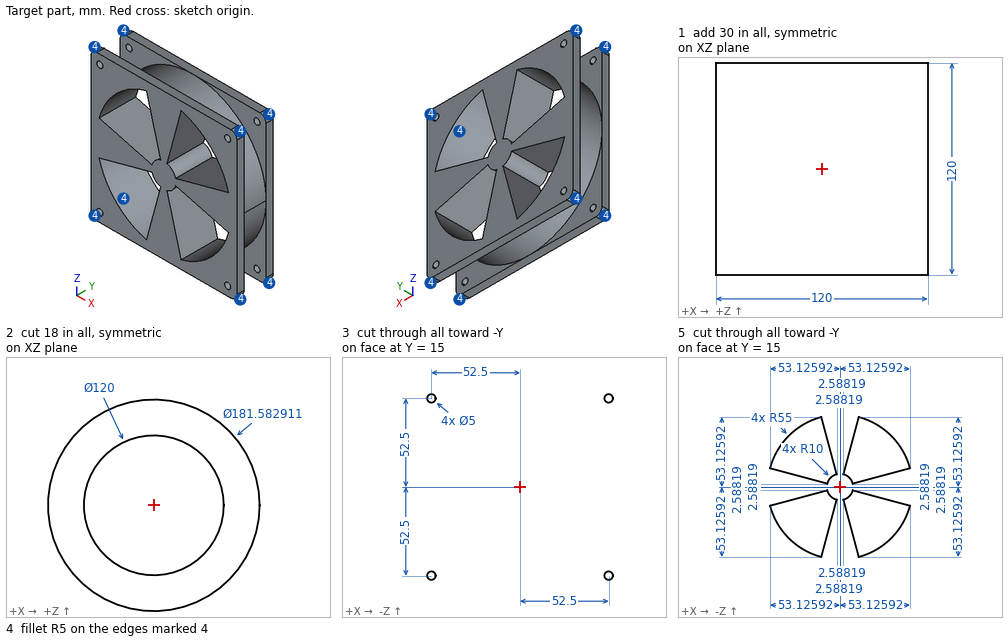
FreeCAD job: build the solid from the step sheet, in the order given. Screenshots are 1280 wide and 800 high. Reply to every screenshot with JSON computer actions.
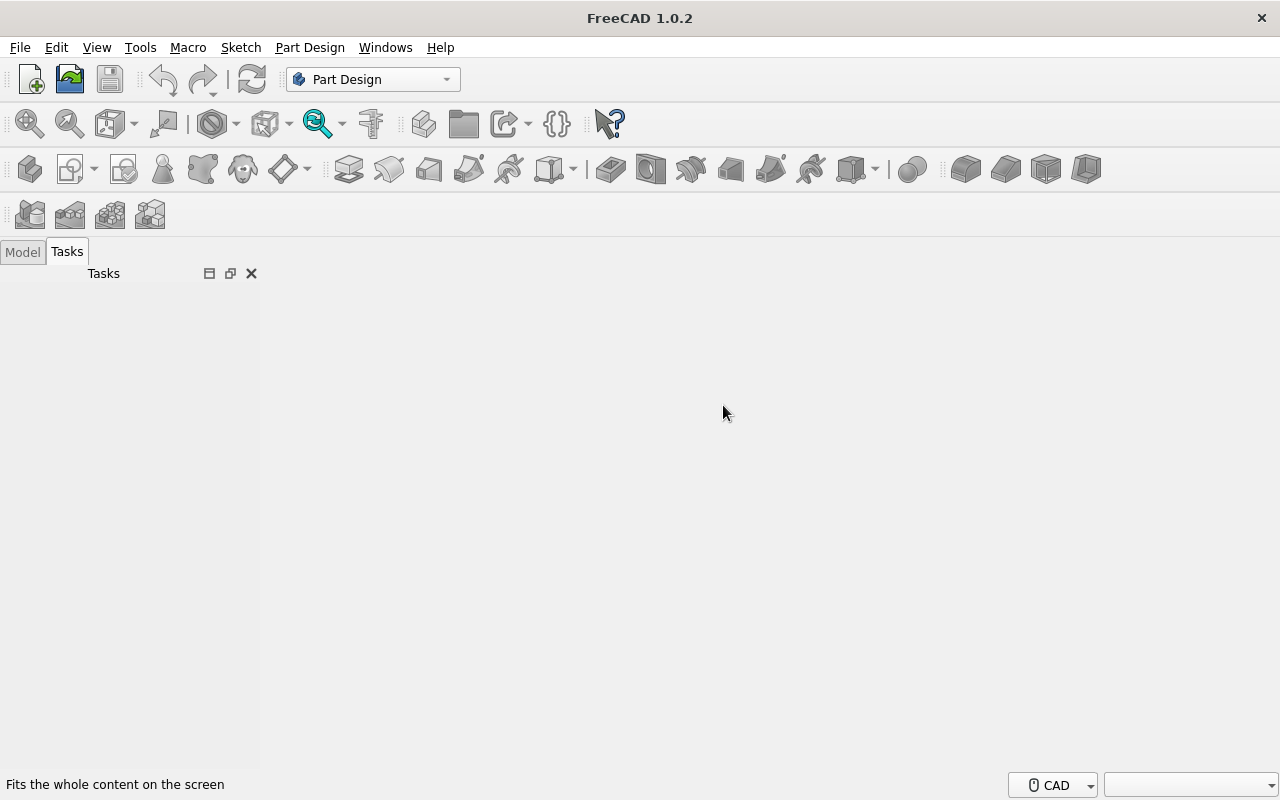
{"action": "left_click", "coordinate": [30, 80]}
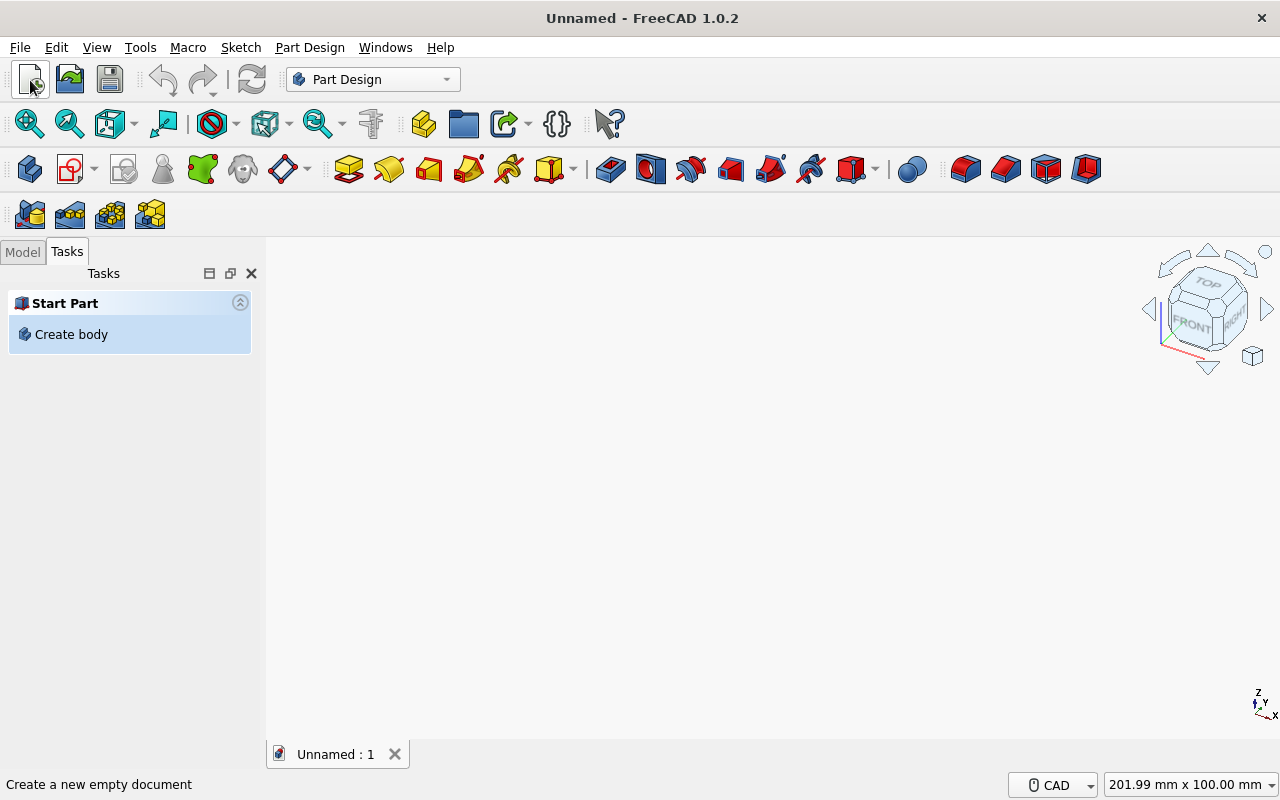
{"action": "left_click", "coordinate": [70, 170]}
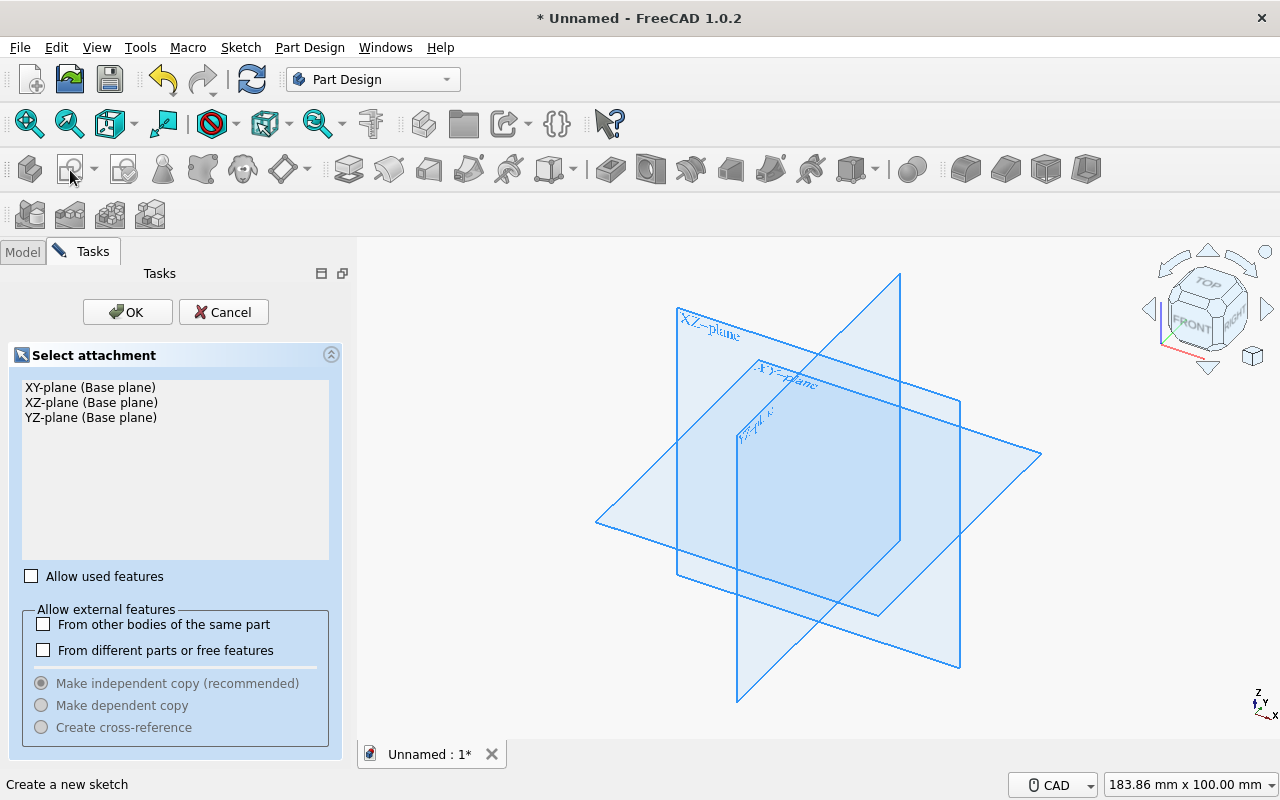
{"action": "left_click", "coordinate": [82, 402]}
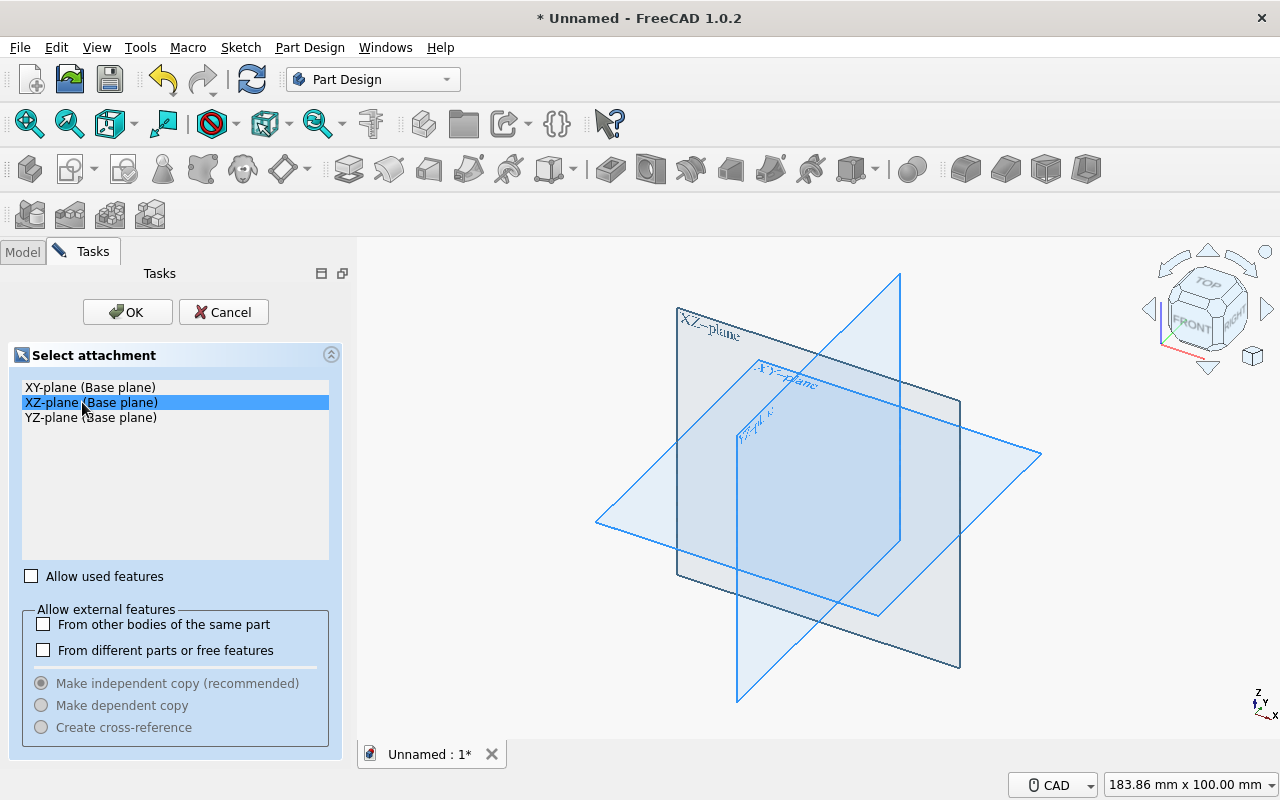
{"action": "left_click", "coordinate": [128, 312]}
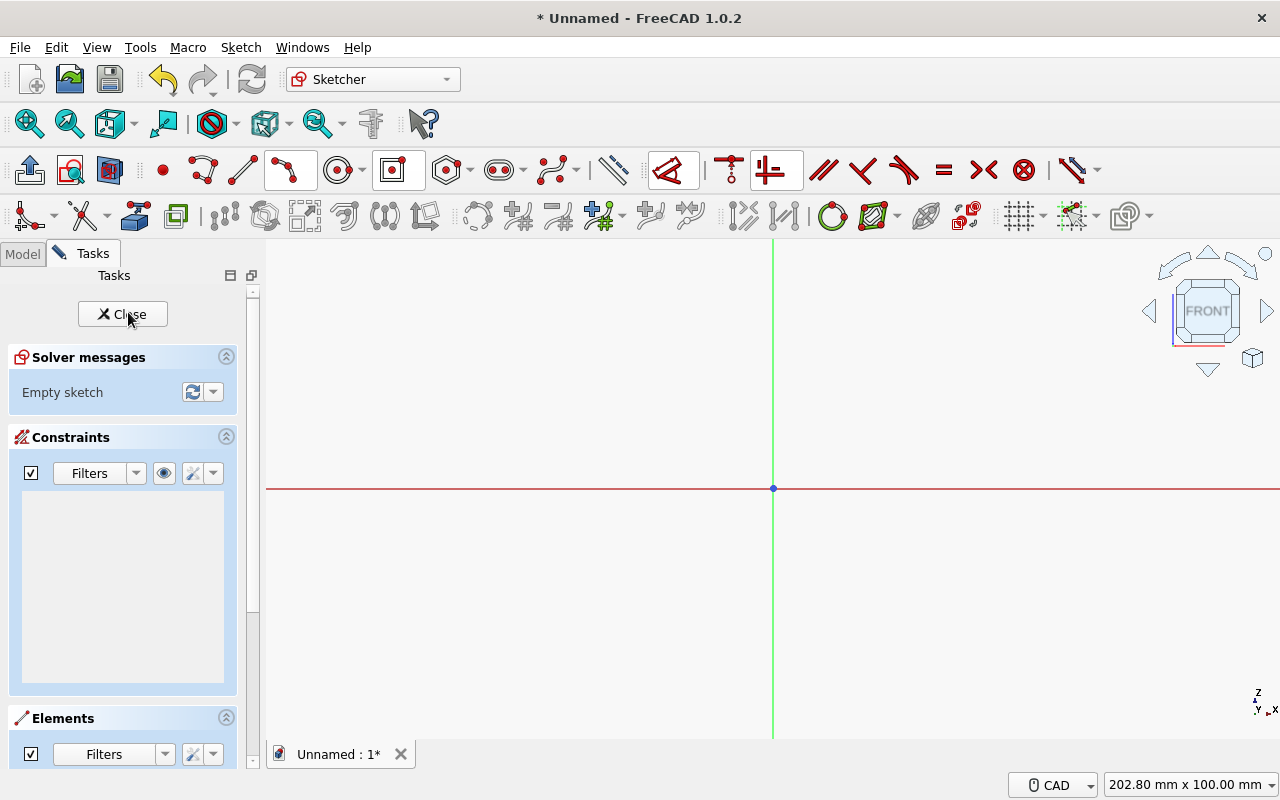
{"action": "scroll", "coordinate": [621, 489], "scroll_direction": "down", "scroll_amount": 3}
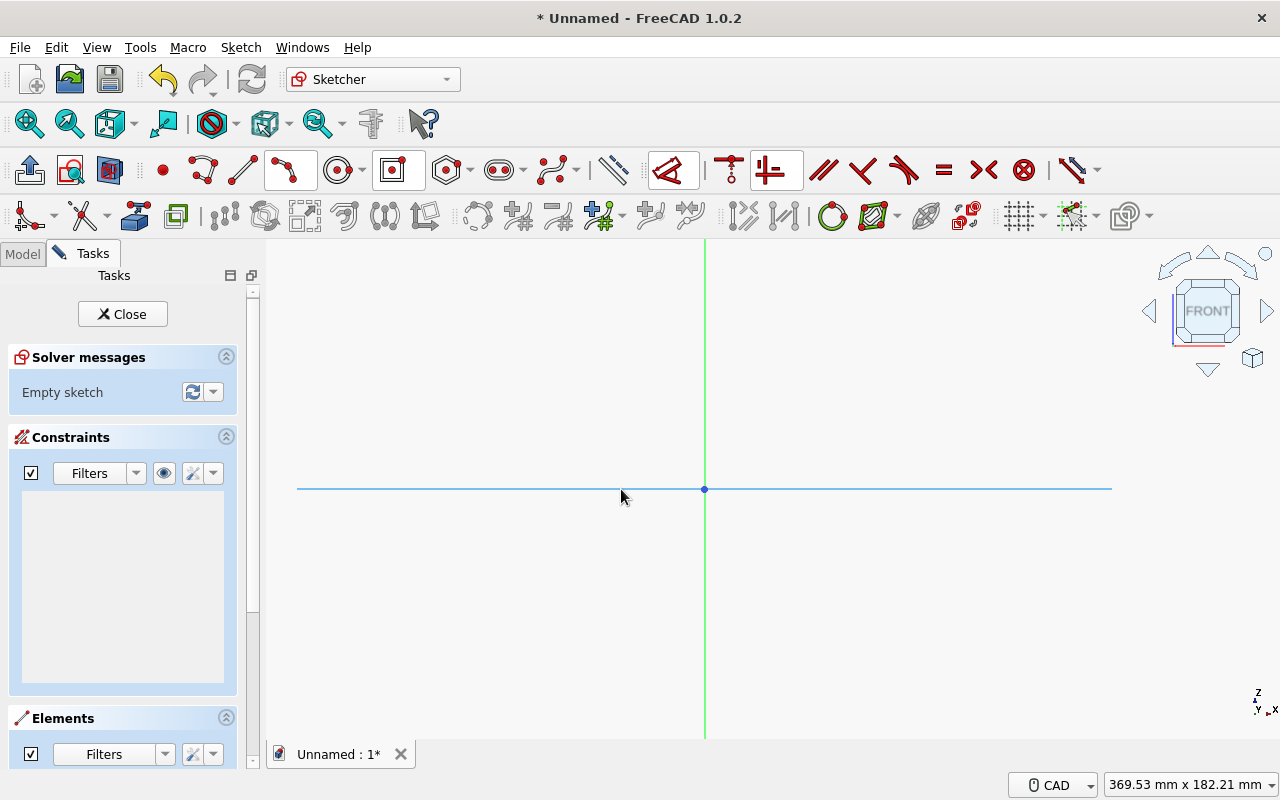
{"action": "left_click", "coordinate": [392, 170]}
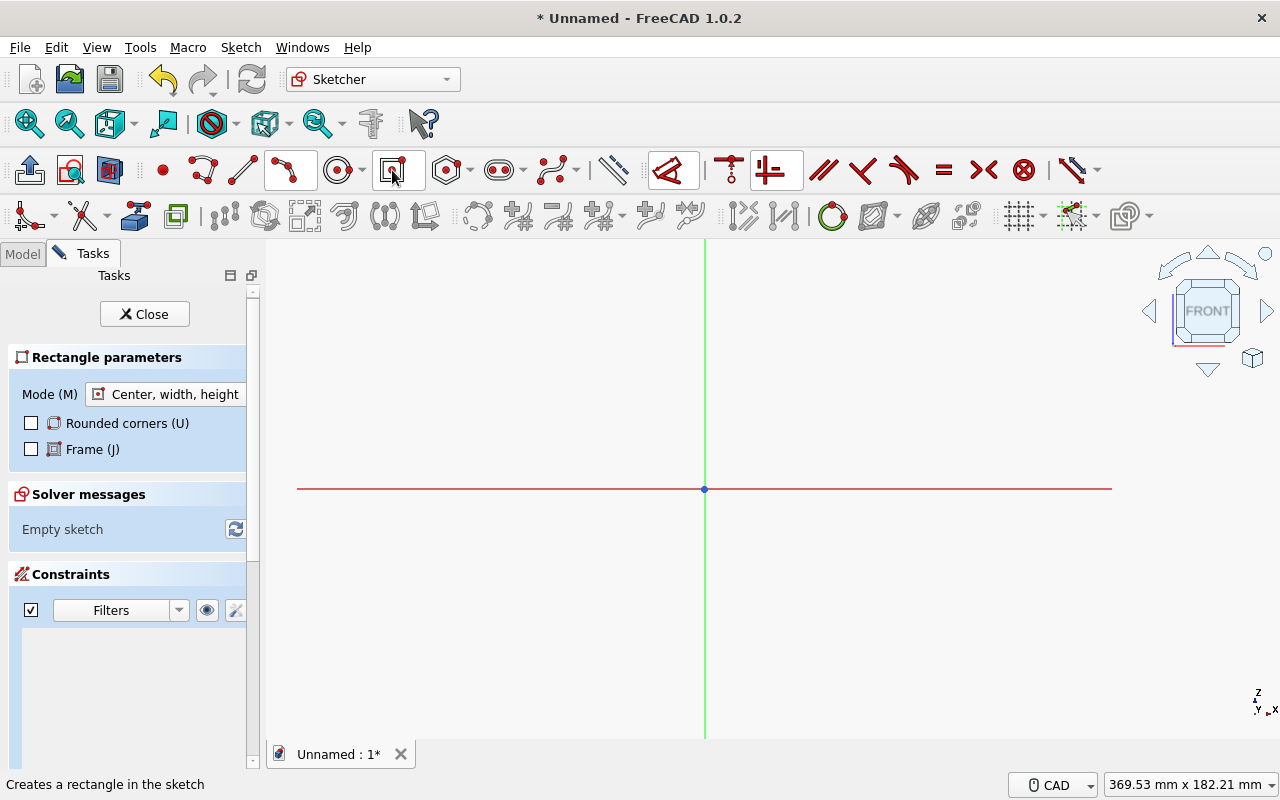
{"action": "left_click", "coordinate": [705, 489]}
{"action": "left_click", "coordinate": [869, 325]}
{"action": "key", "text": "Escape"}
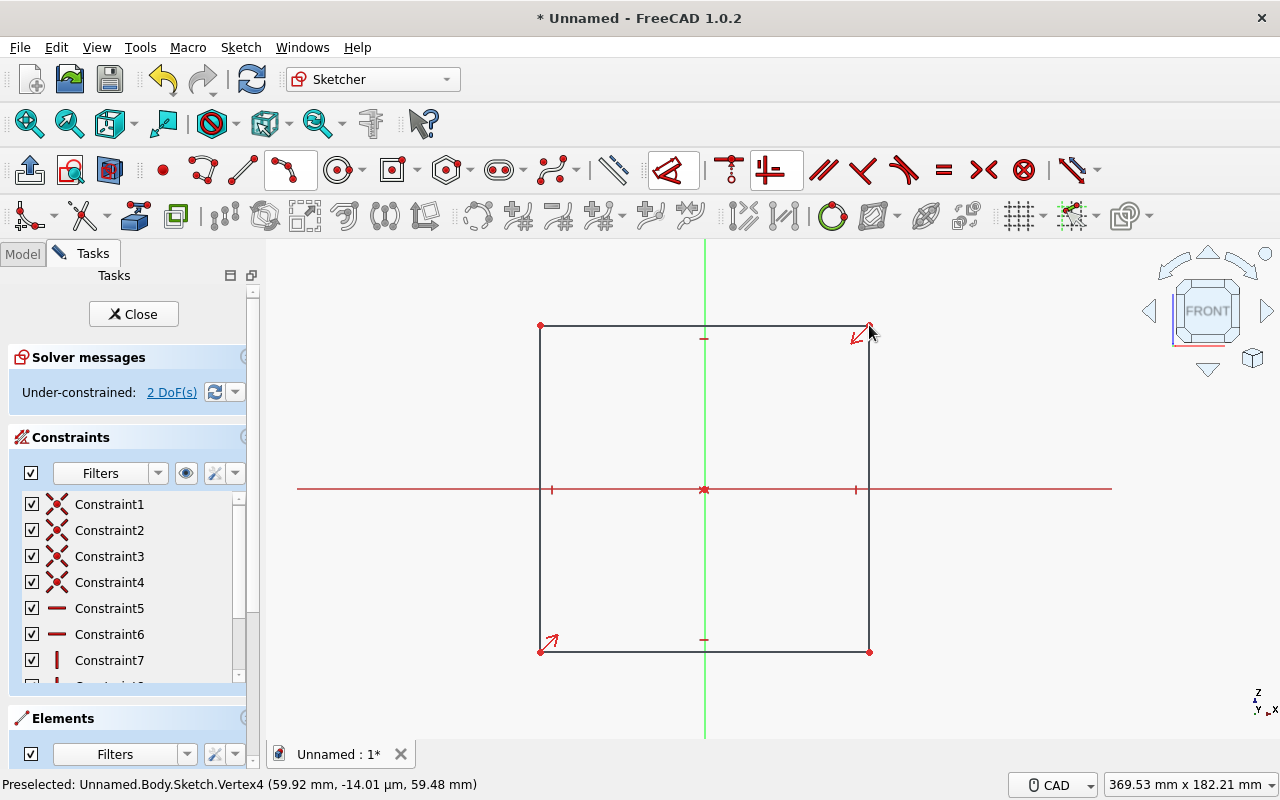
{"action": "left_click", "coordinate": [639, 652]}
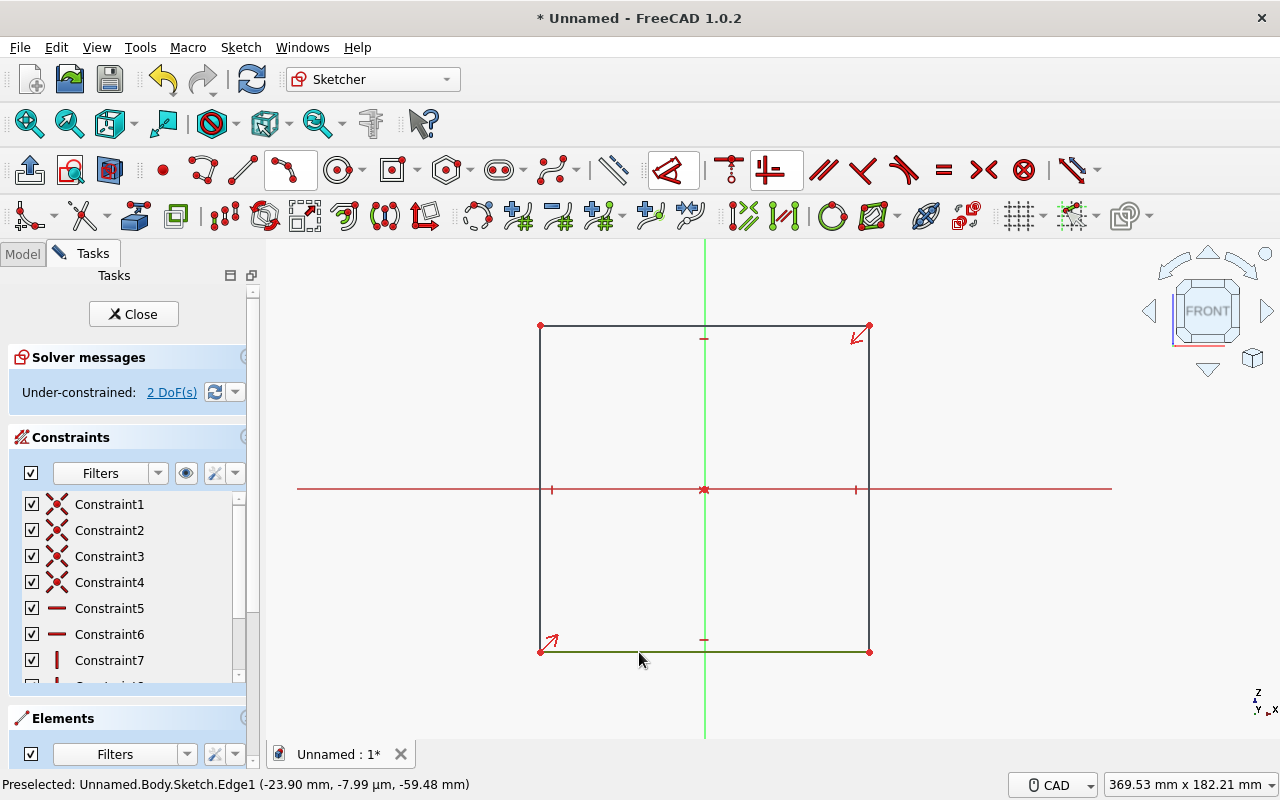
{"action": "left_click", "coordinate": [694, 170]}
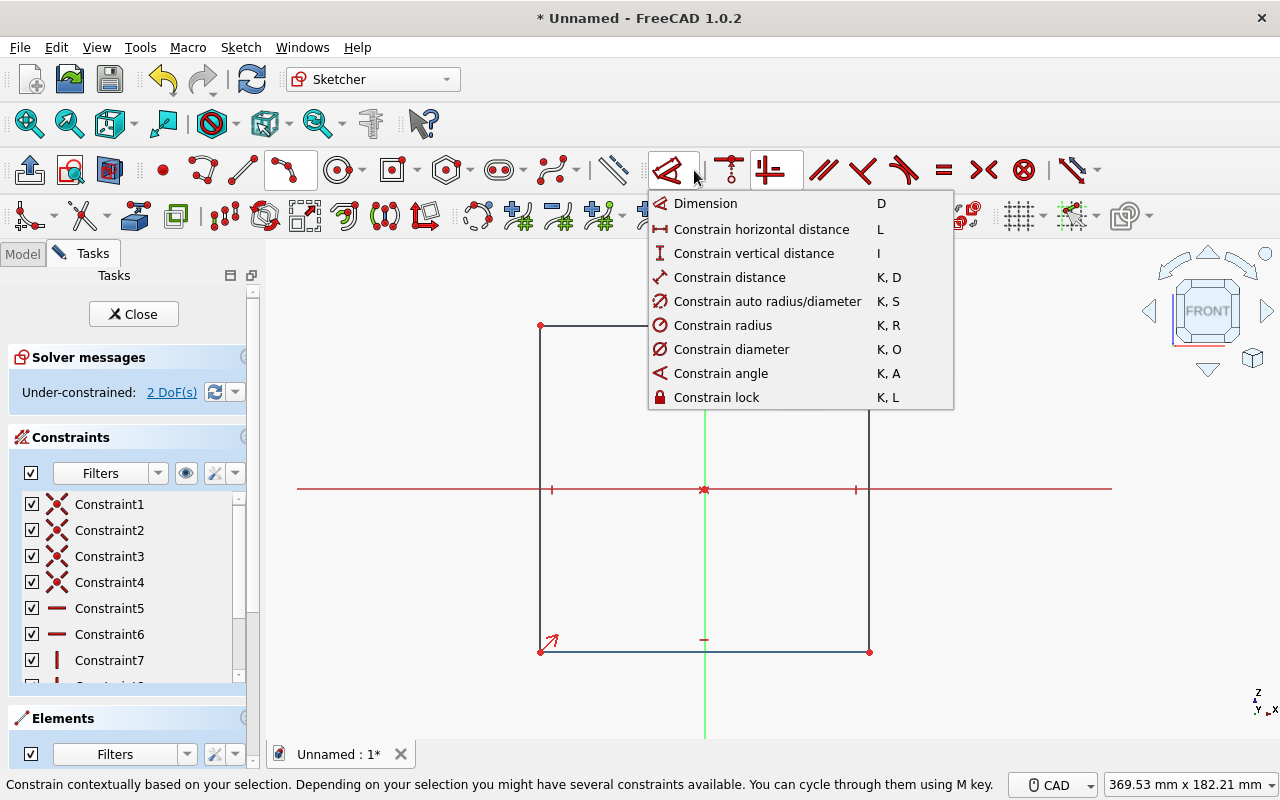
{"action": "left_click", "coordinate": [801, 229]}